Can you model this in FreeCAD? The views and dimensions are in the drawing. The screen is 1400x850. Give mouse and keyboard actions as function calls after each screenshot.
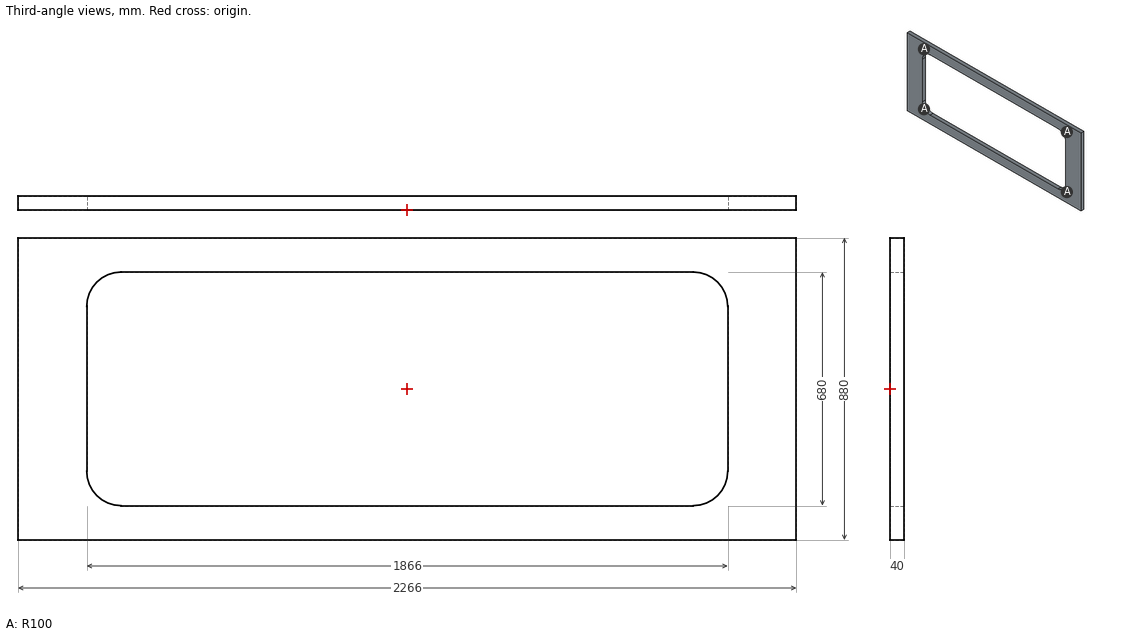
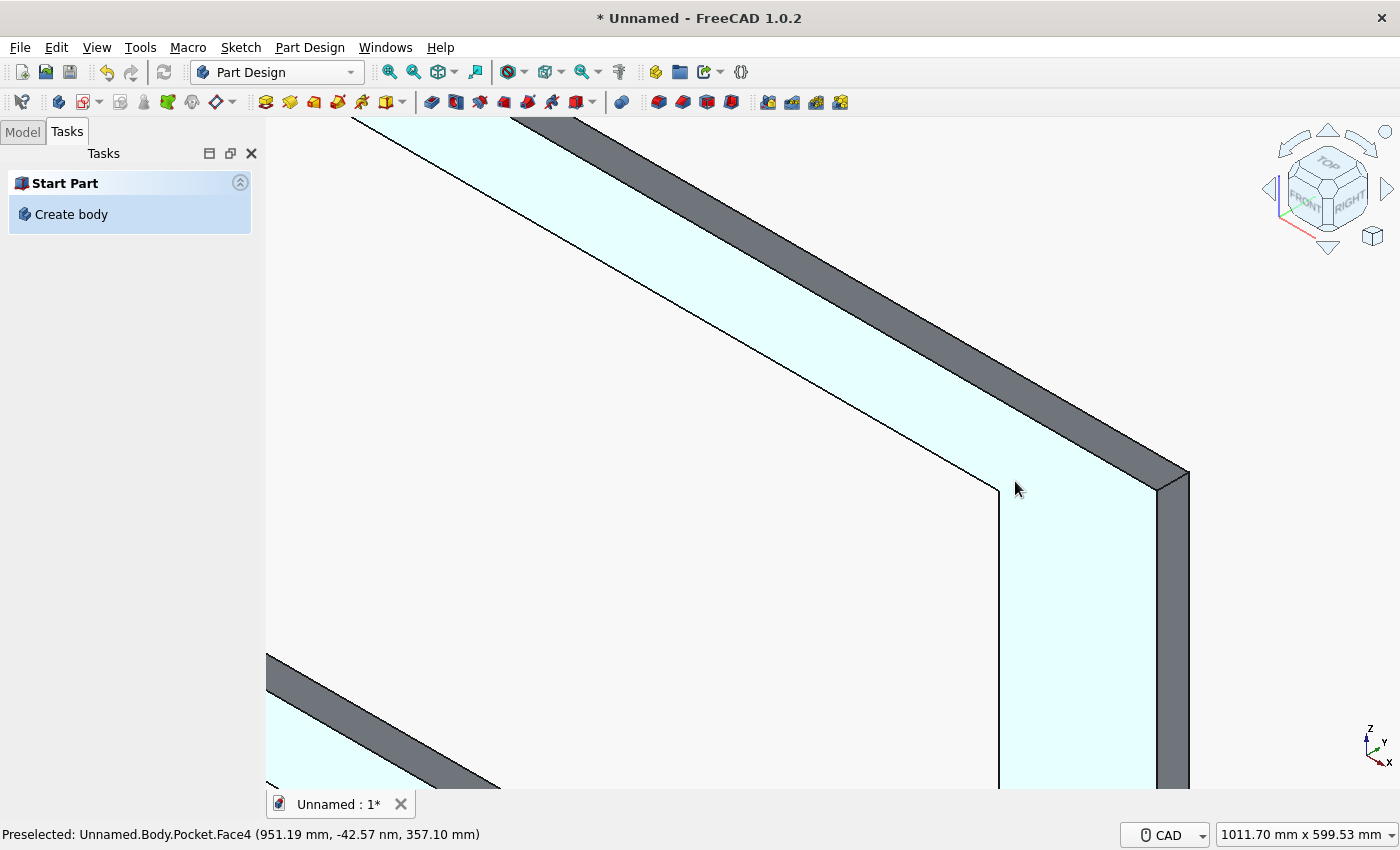
click(390, 72)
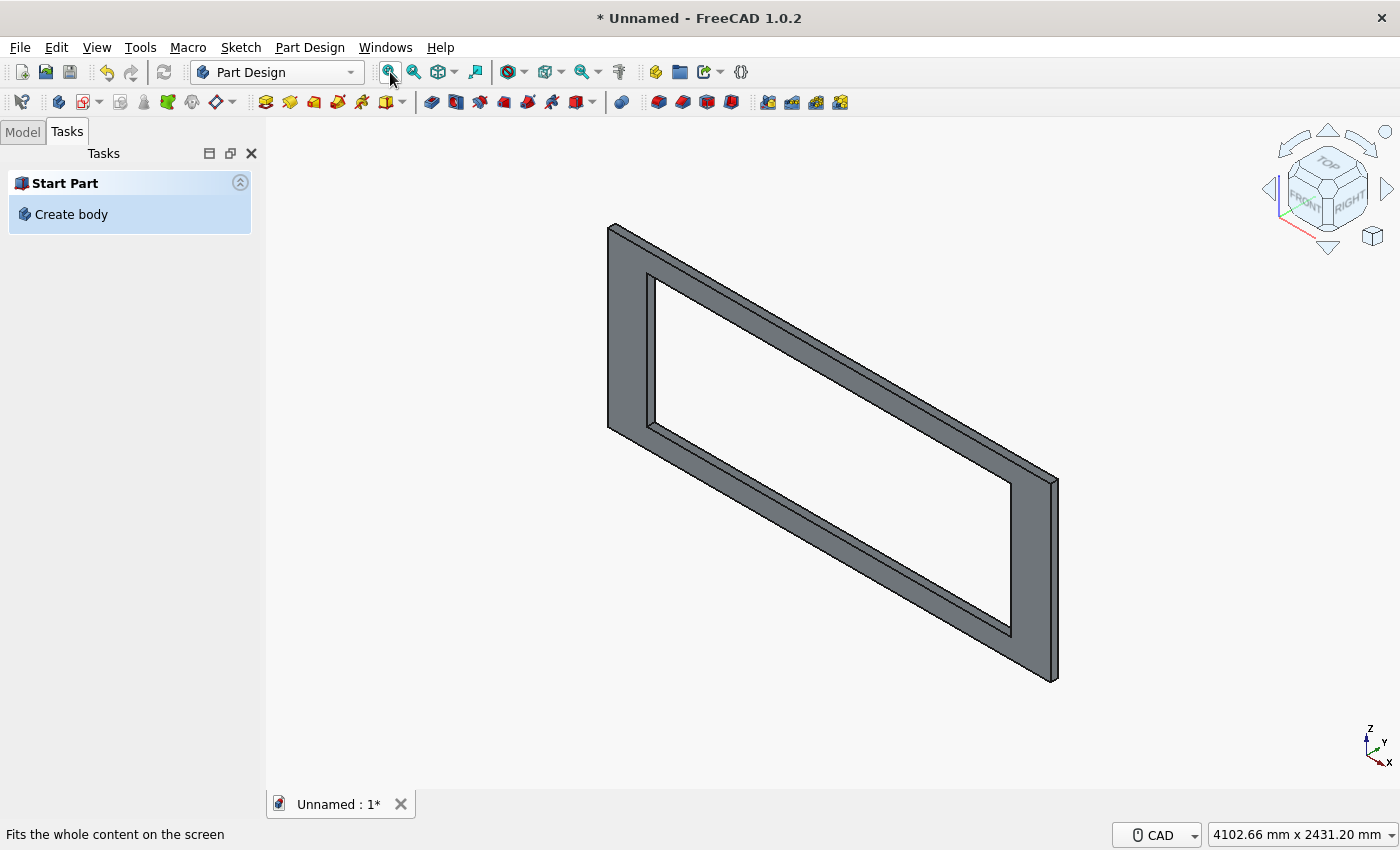
key(2)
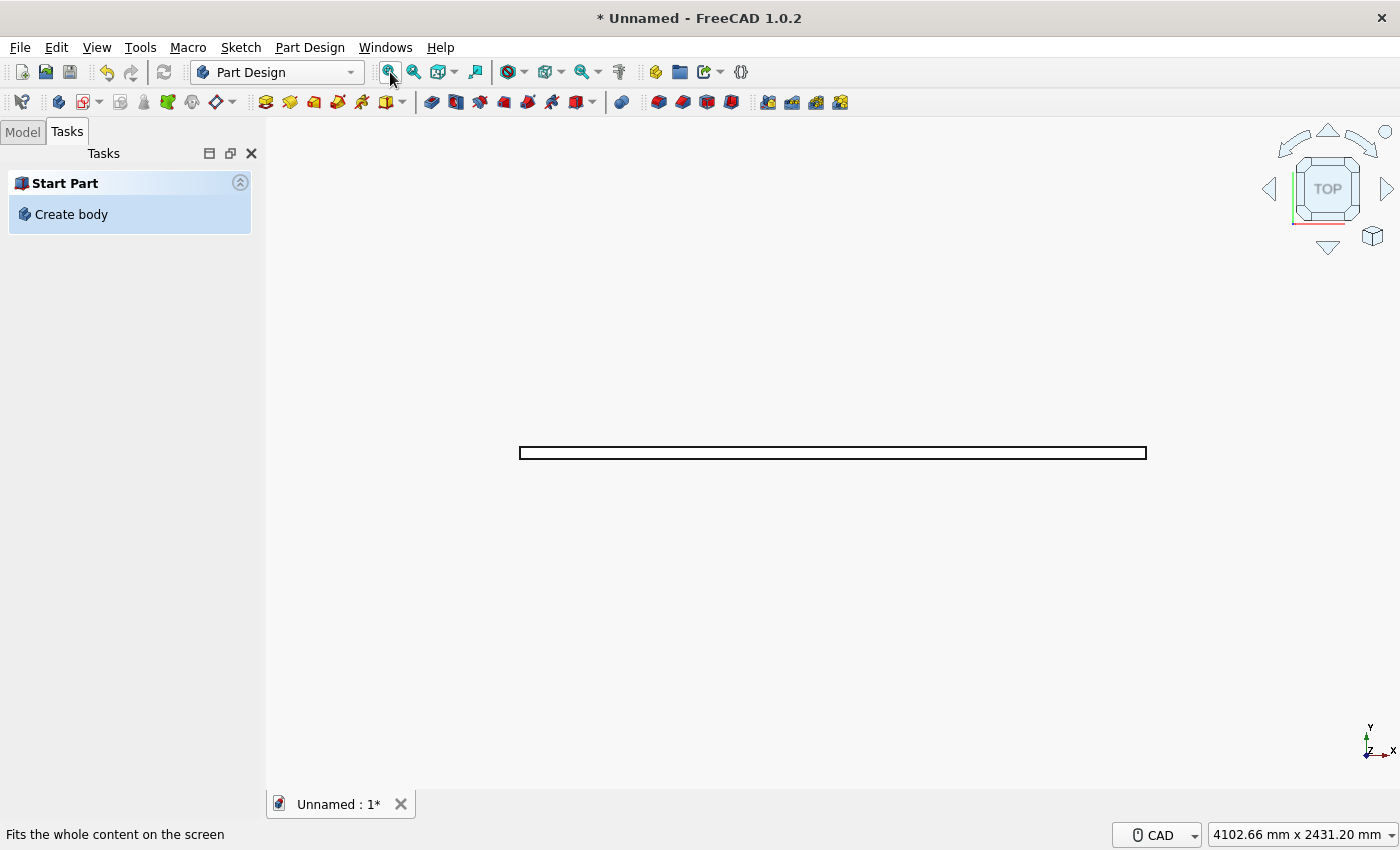
scroll(1091, 452, up, 7)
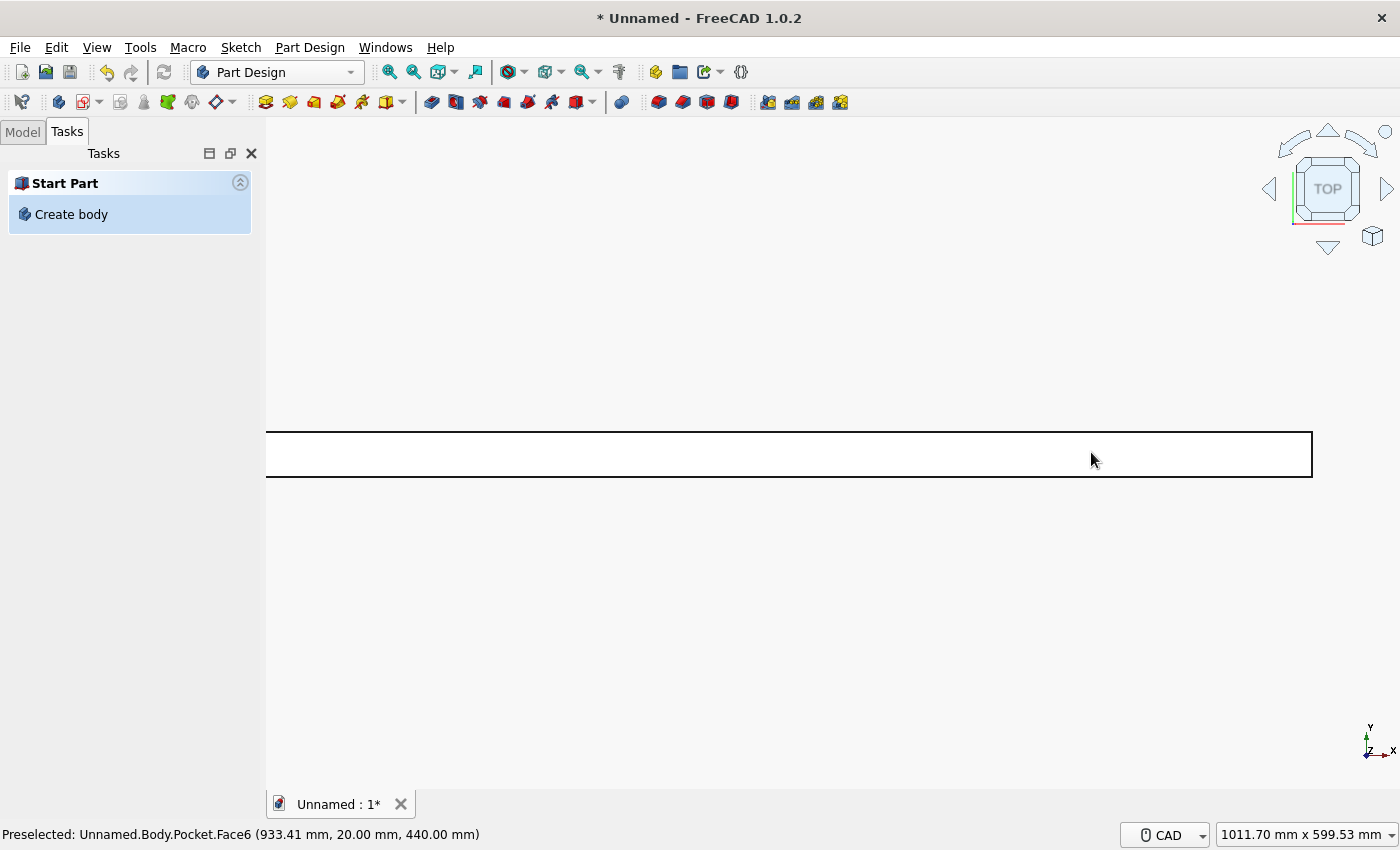
click(390, 72)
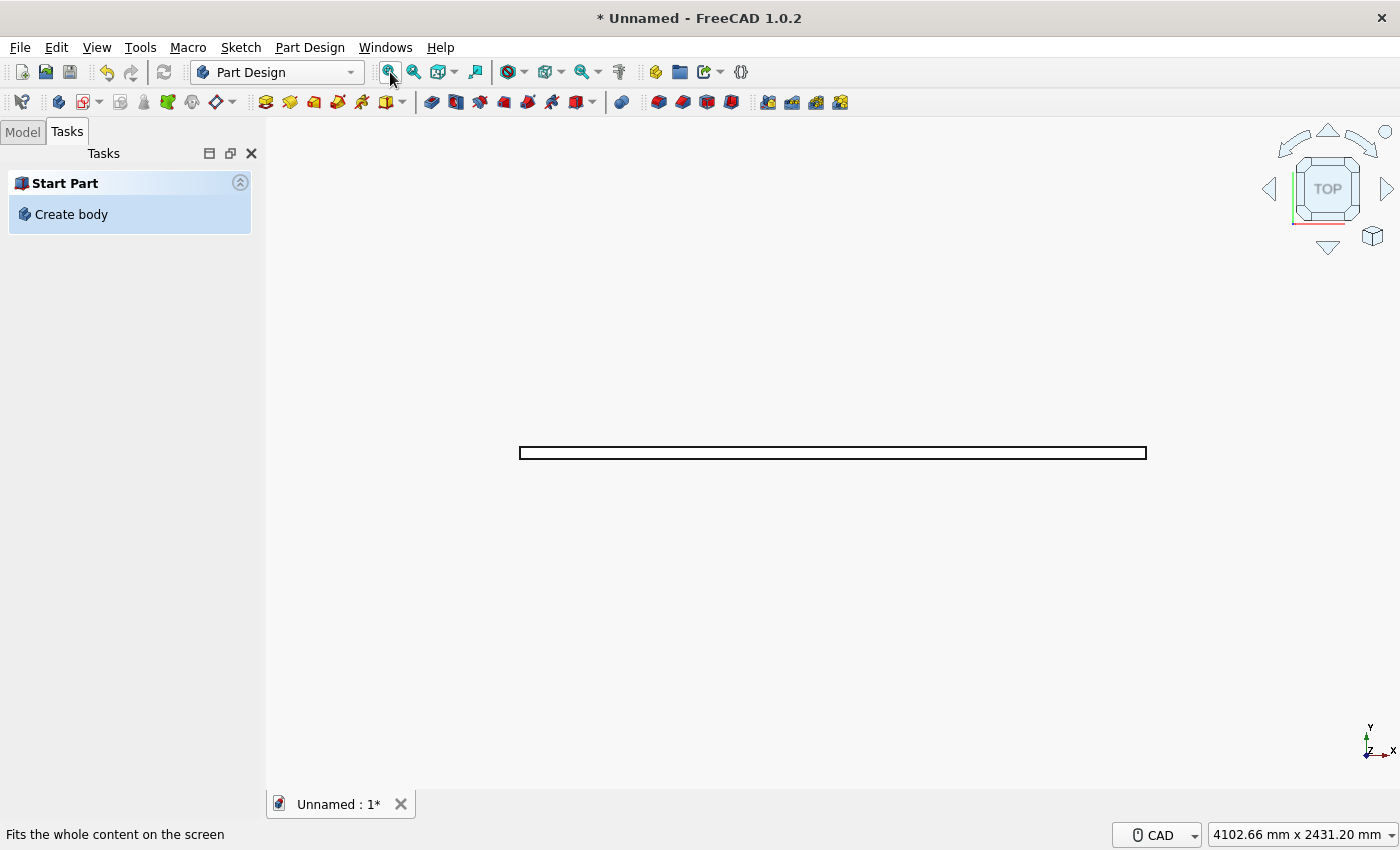
key(1)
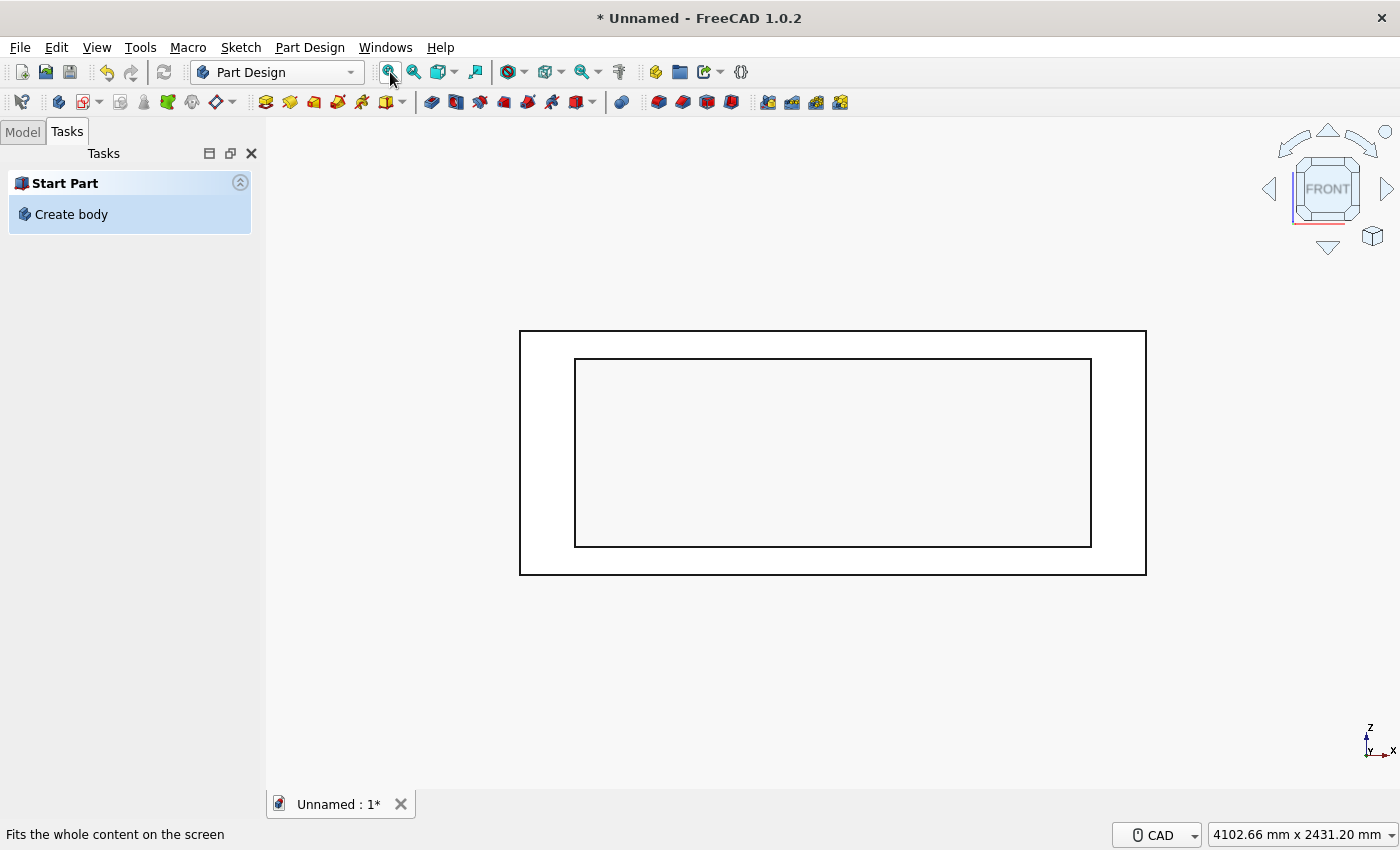
scroll(1091, 358, up, 7)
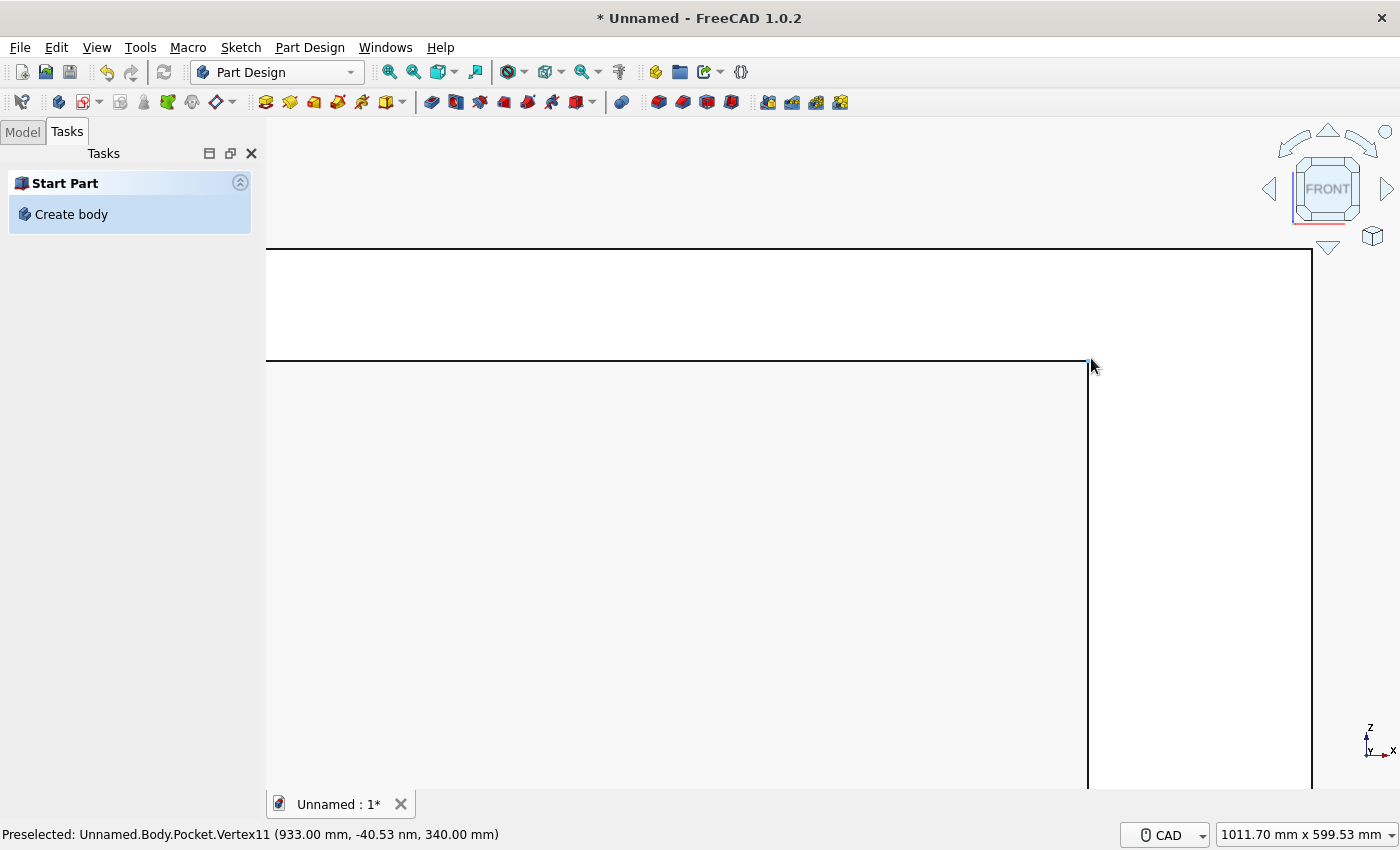
key(v)
key(f)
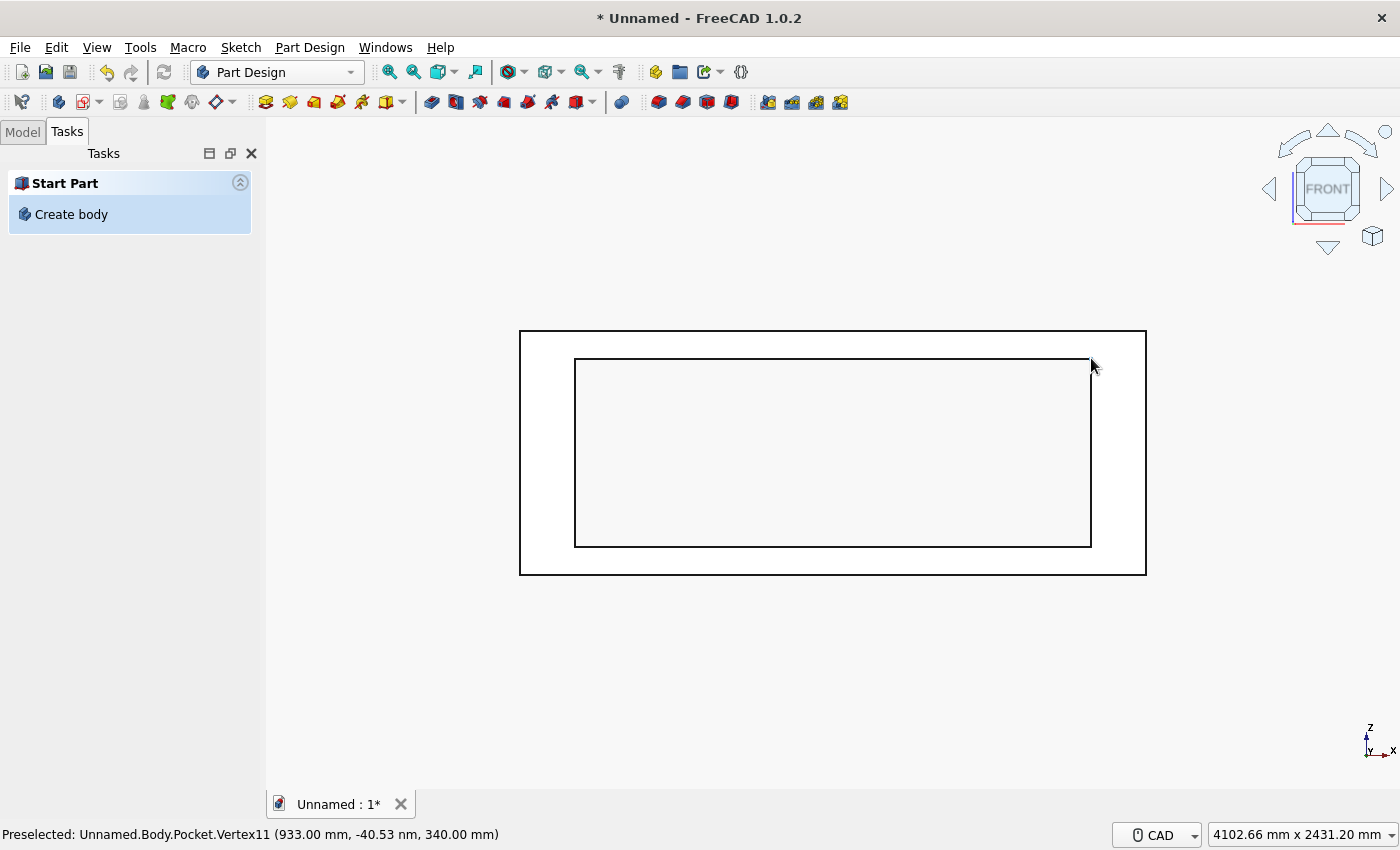
key(3)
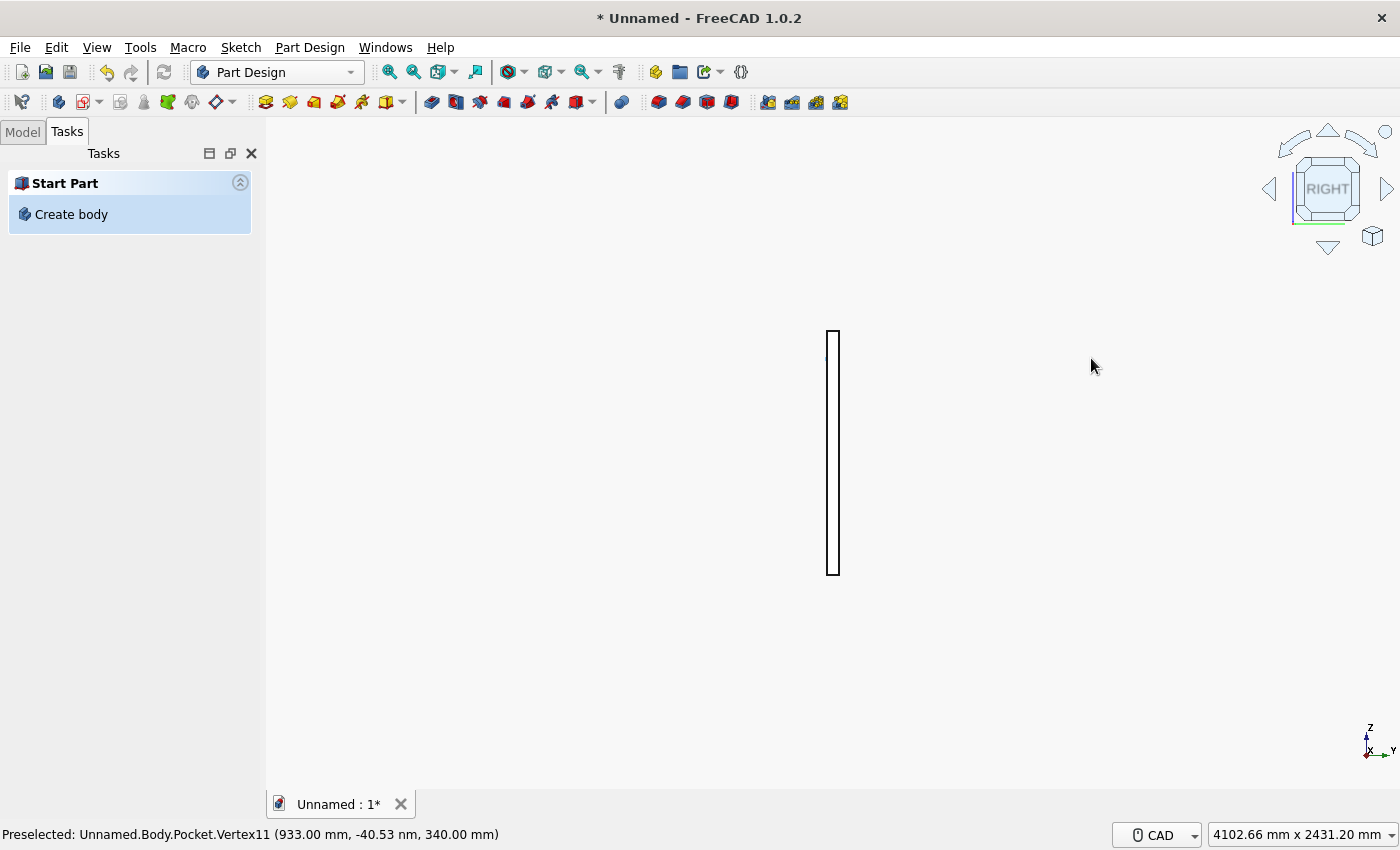
key(v)
key(f)